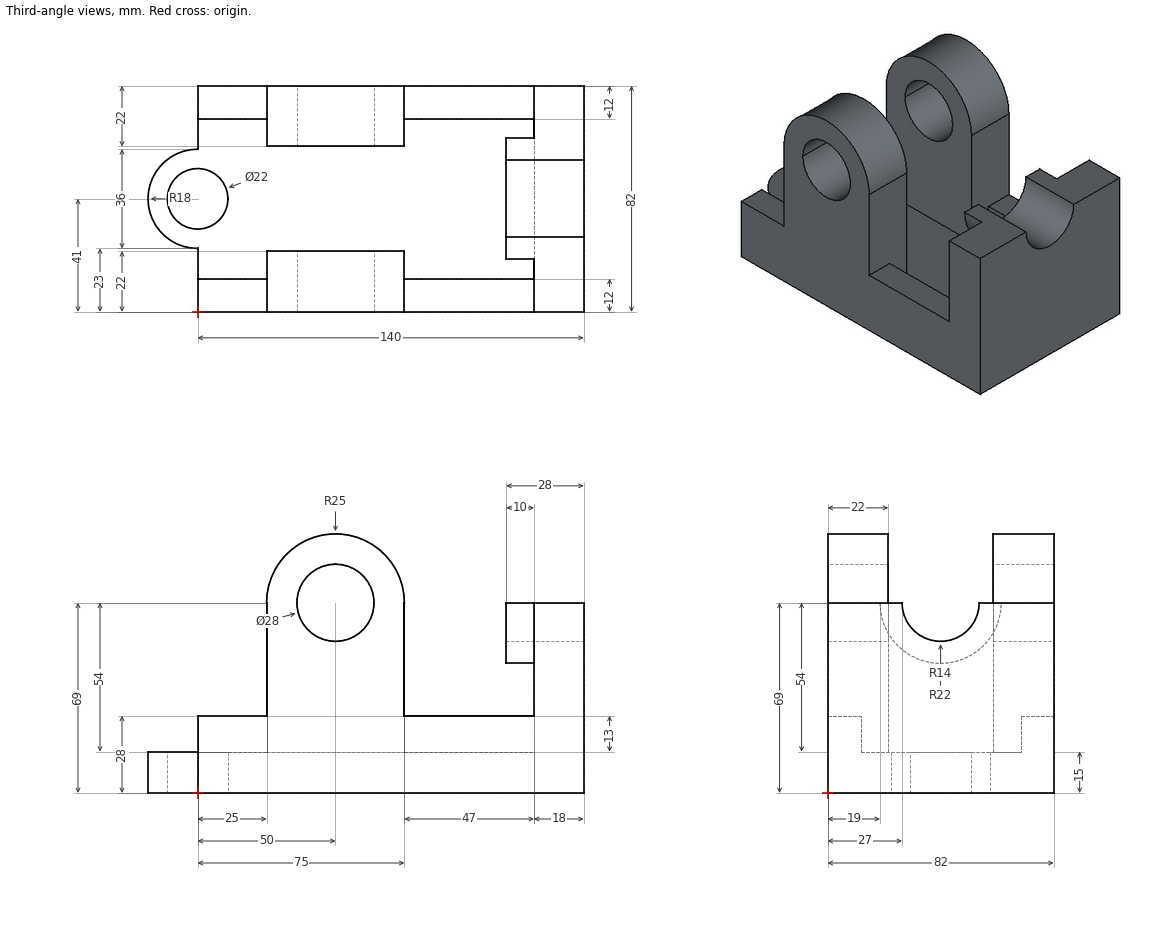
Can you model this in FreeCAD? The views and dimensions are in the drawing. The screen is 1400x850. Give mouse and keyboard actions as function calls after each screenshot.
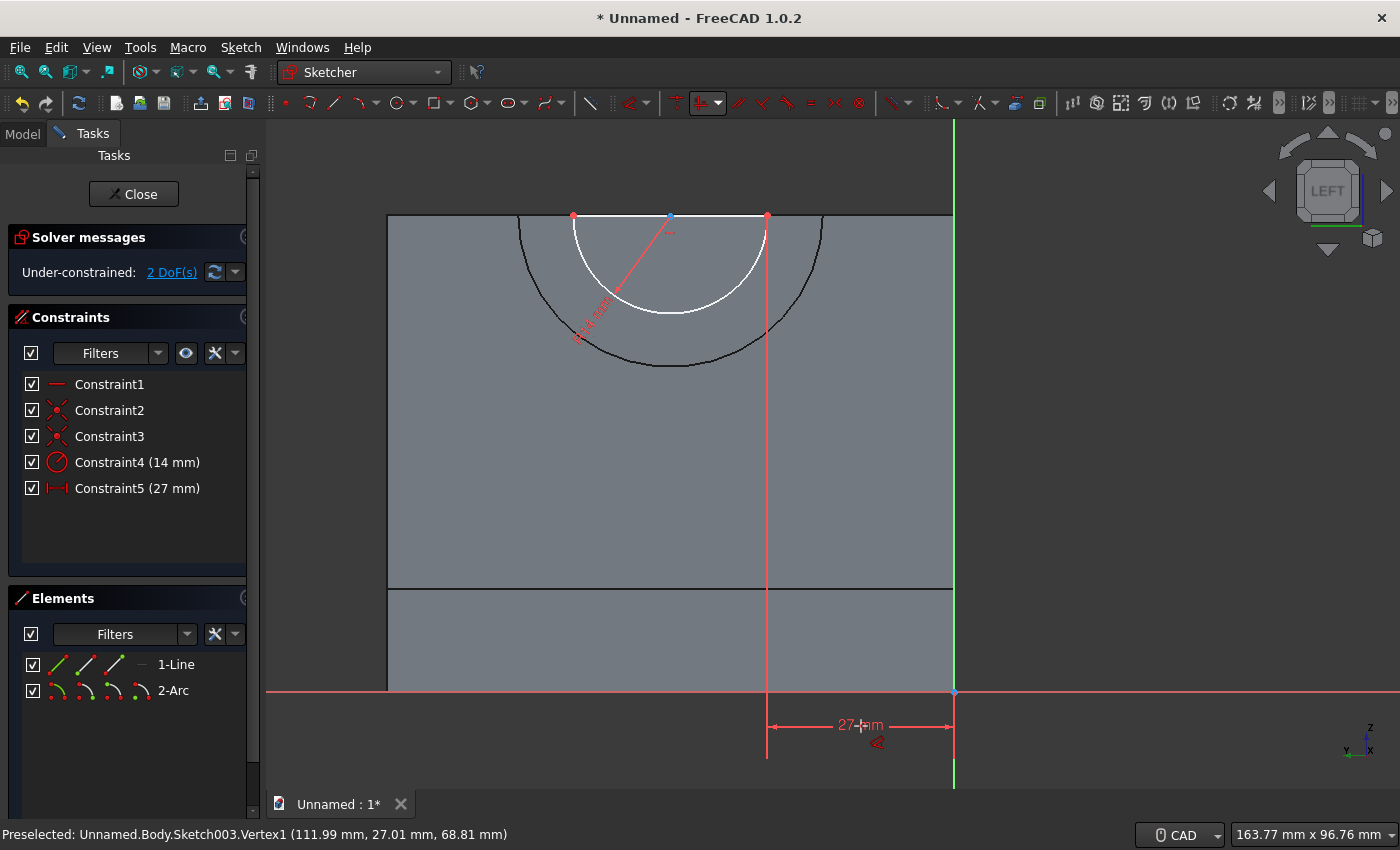
click(767, 216)
click(988, 454)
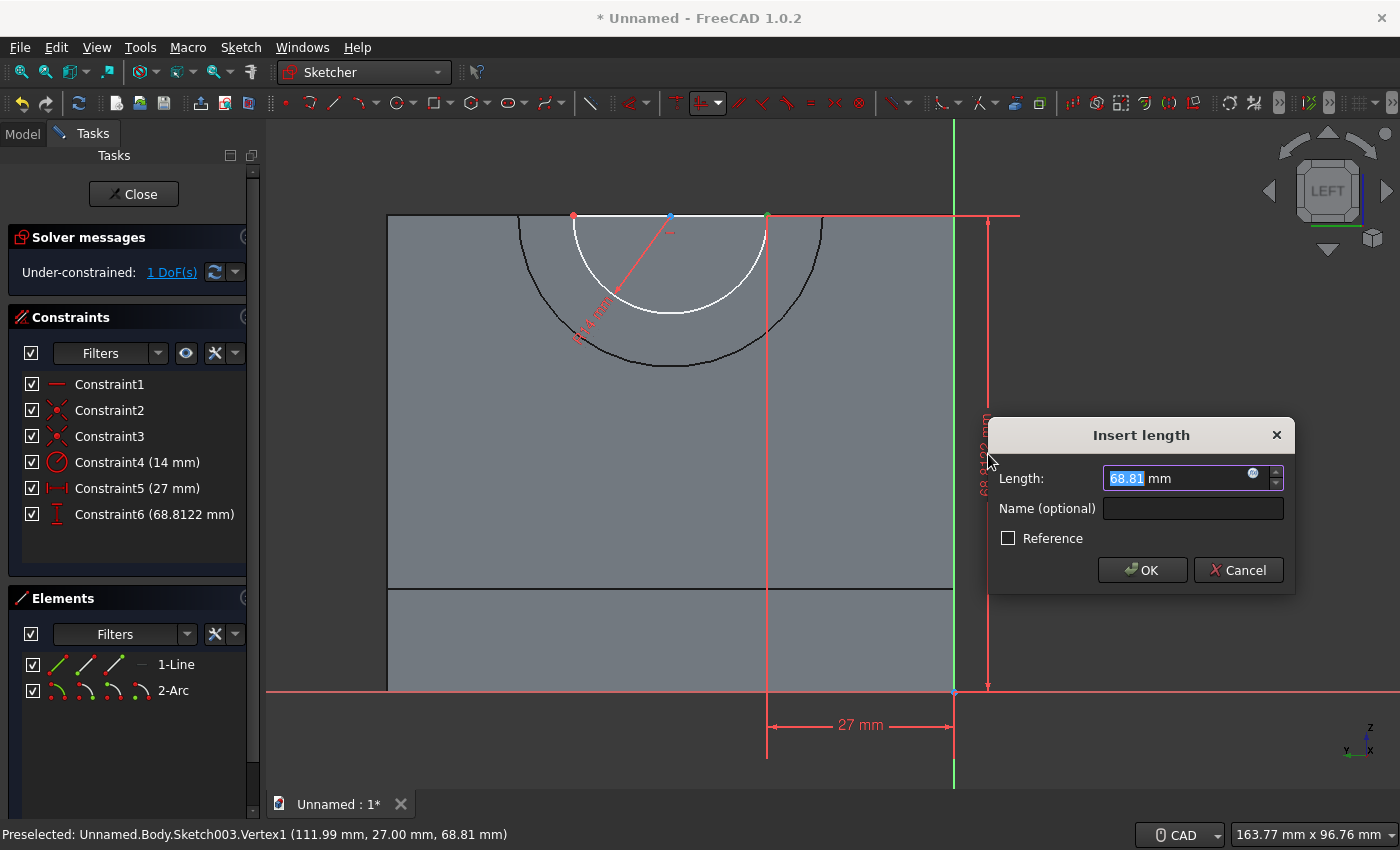
text(69)
key(Return)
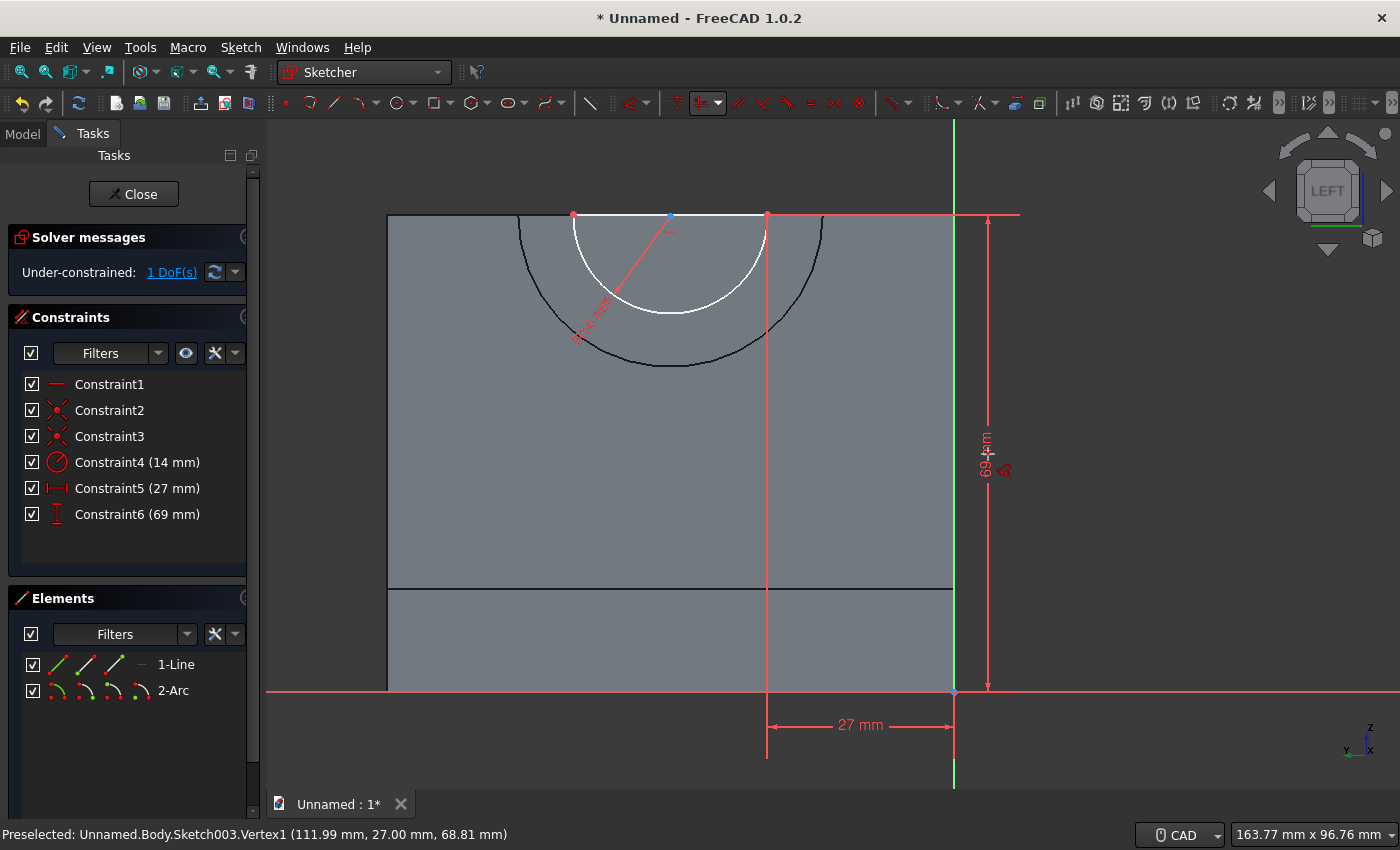
click(671, 216)
click(988, 345)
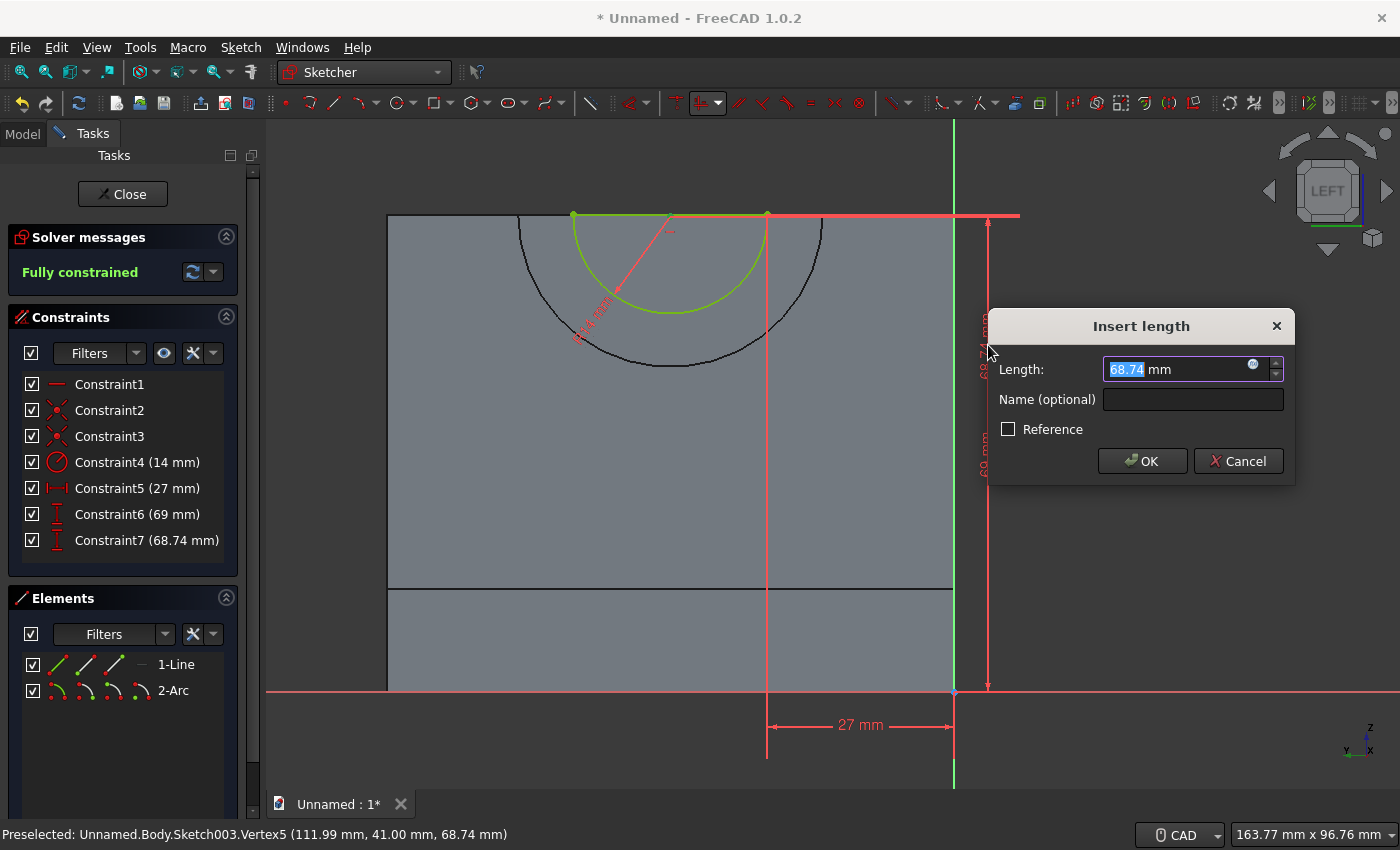
text(69)
key(Return)
key(Escape)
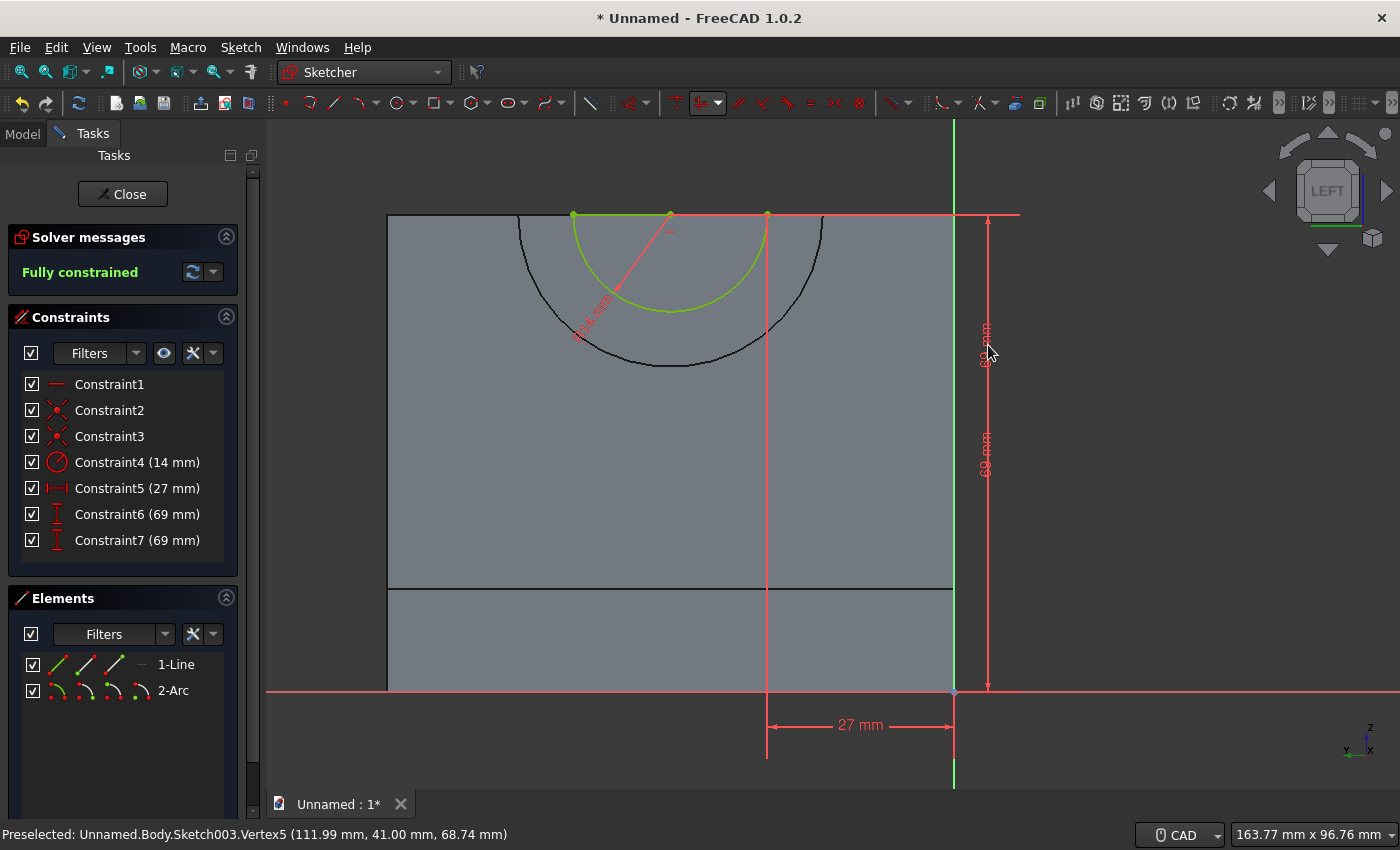
click(123, 194)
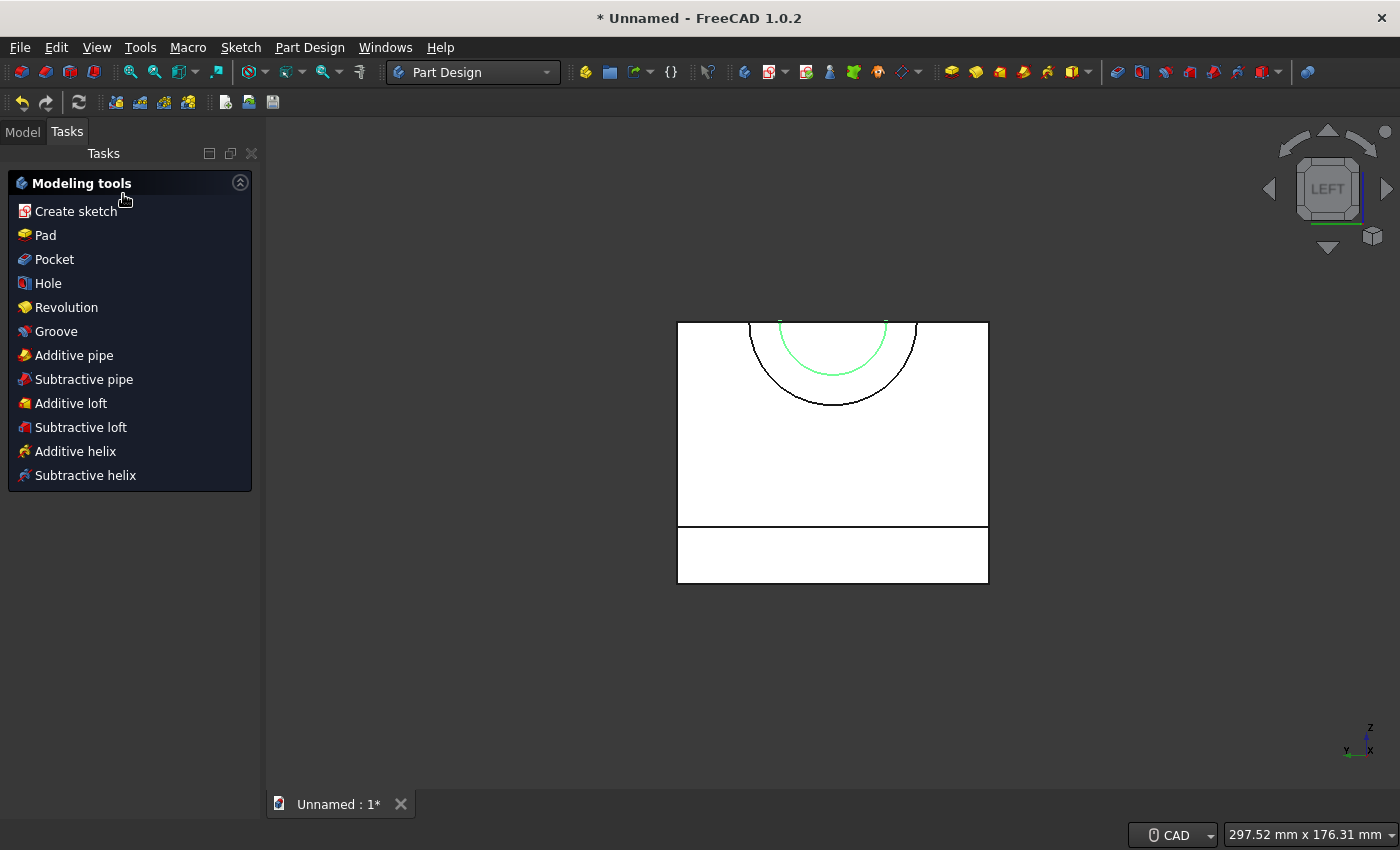
click(1118, 72)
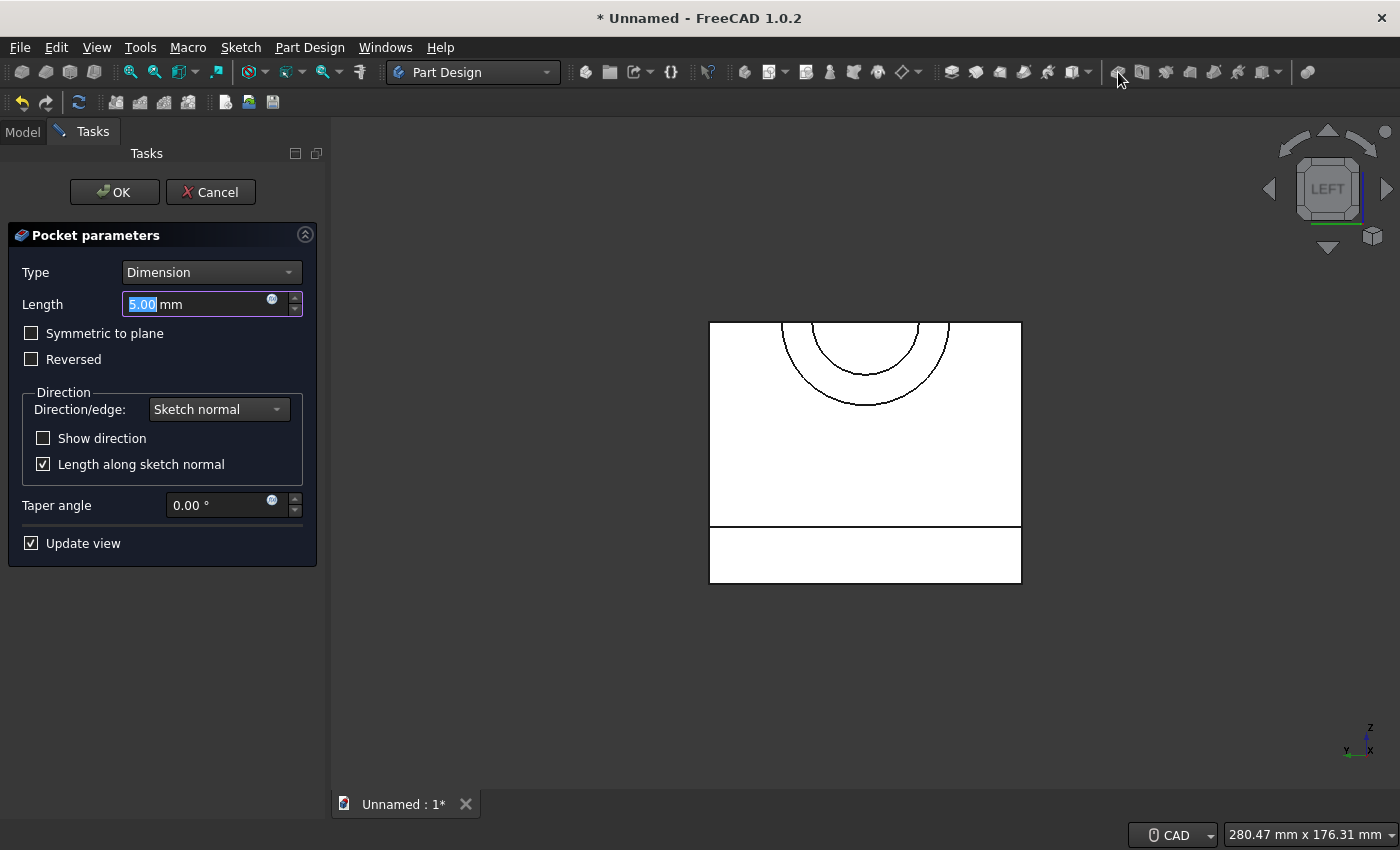
text(28)
key(Tab)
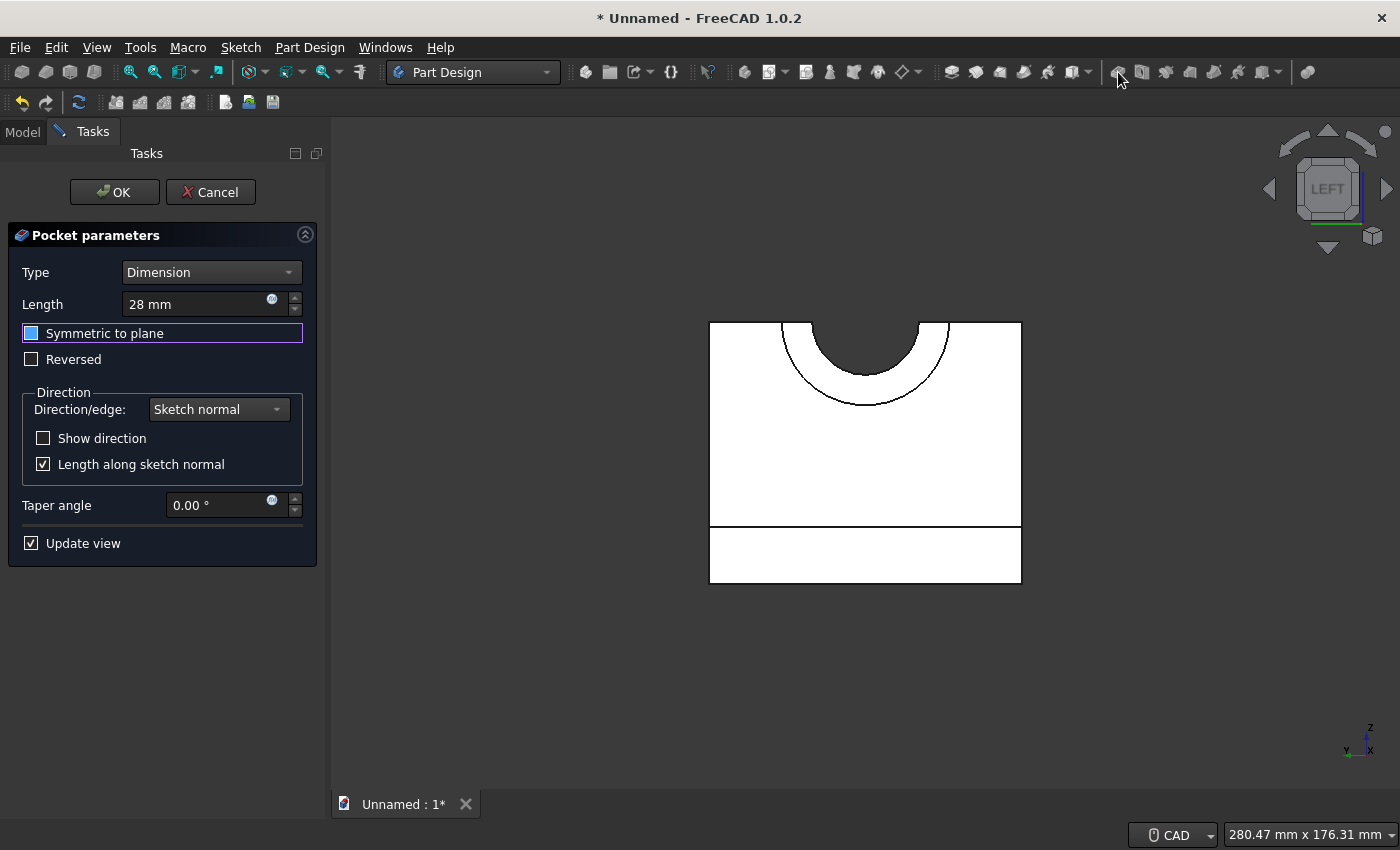
click(115, 192)